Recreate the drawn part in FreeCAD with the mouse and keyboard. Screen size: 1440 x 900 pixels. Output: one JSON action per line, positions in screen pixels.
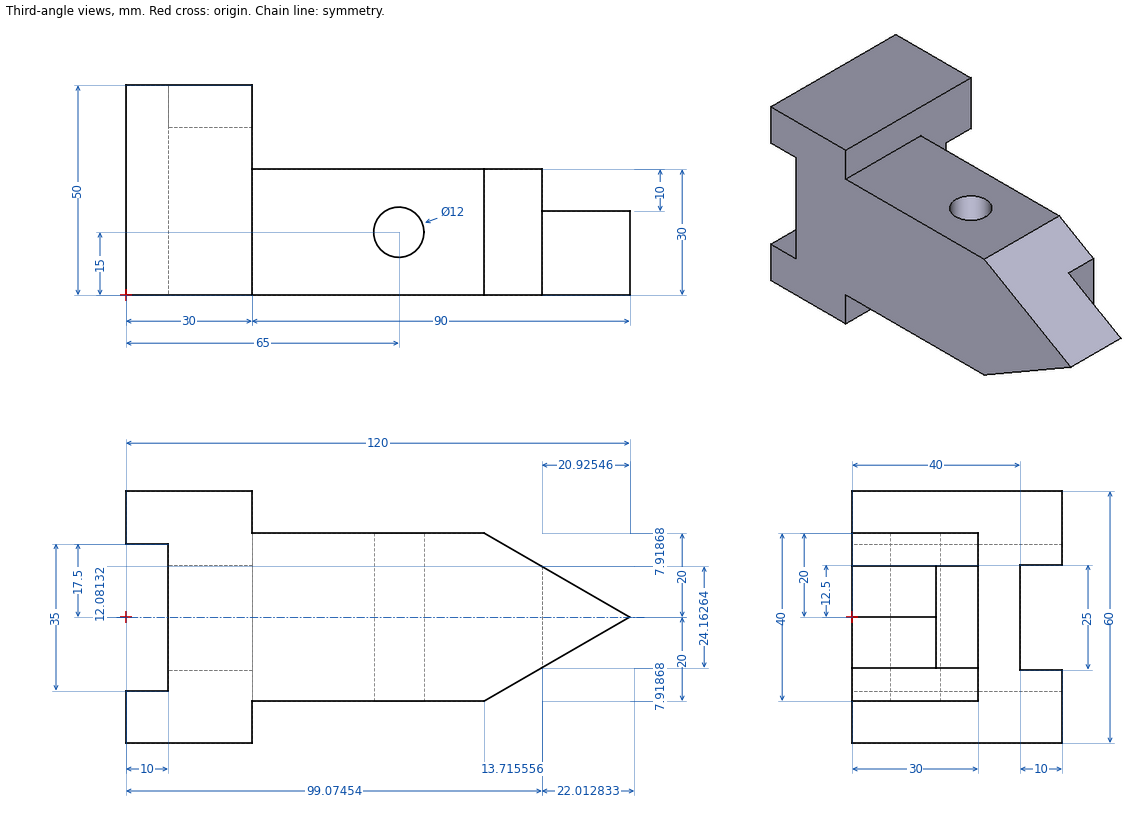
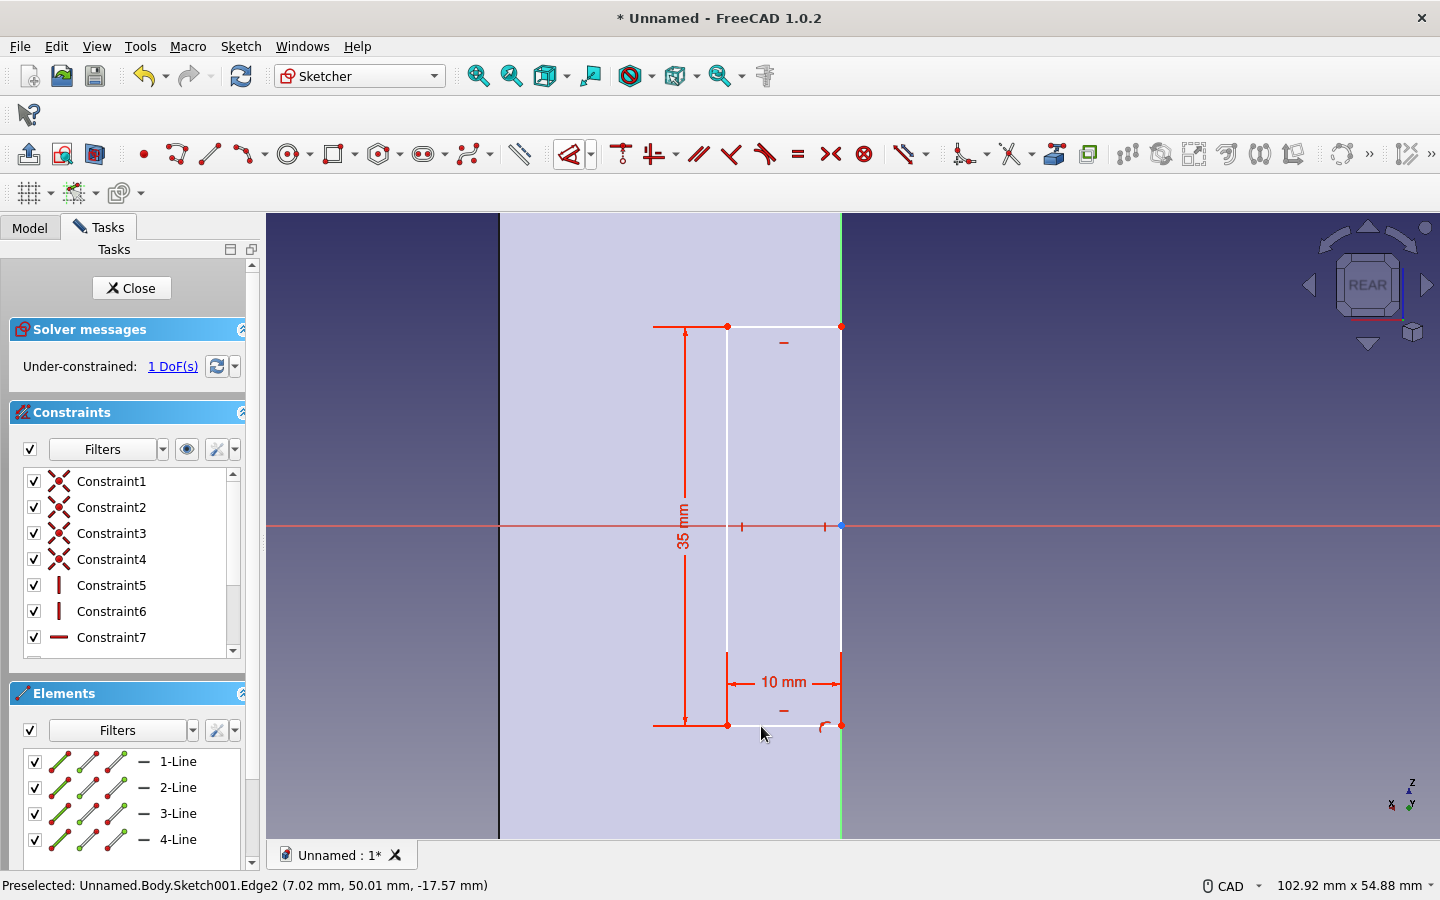
{"action": "left_click", "coordinate": [727, 327]}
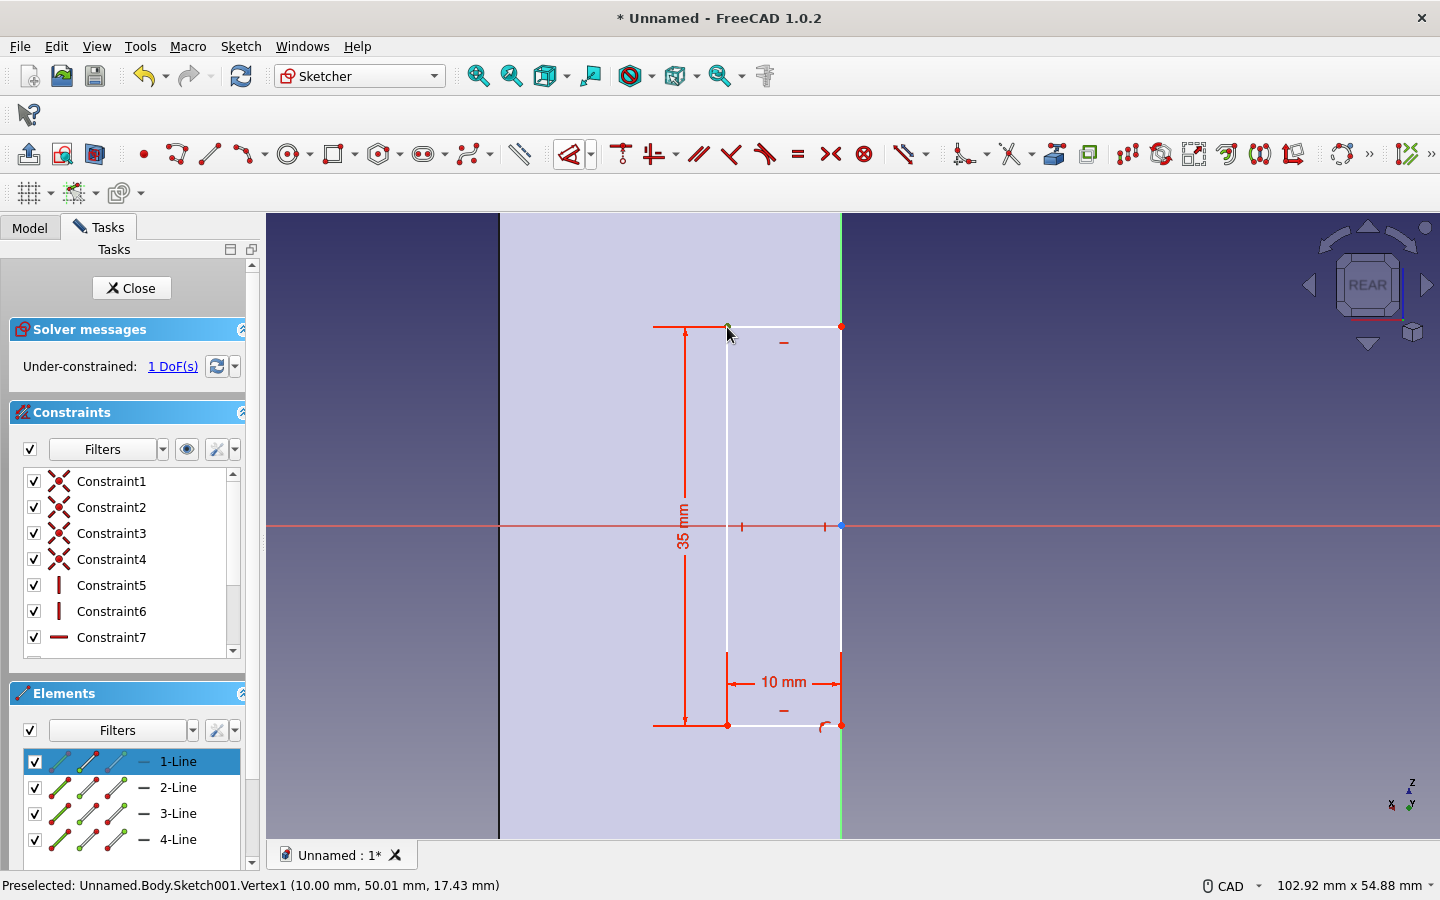
{"action": "left_click", "coordinate": [590, 154]}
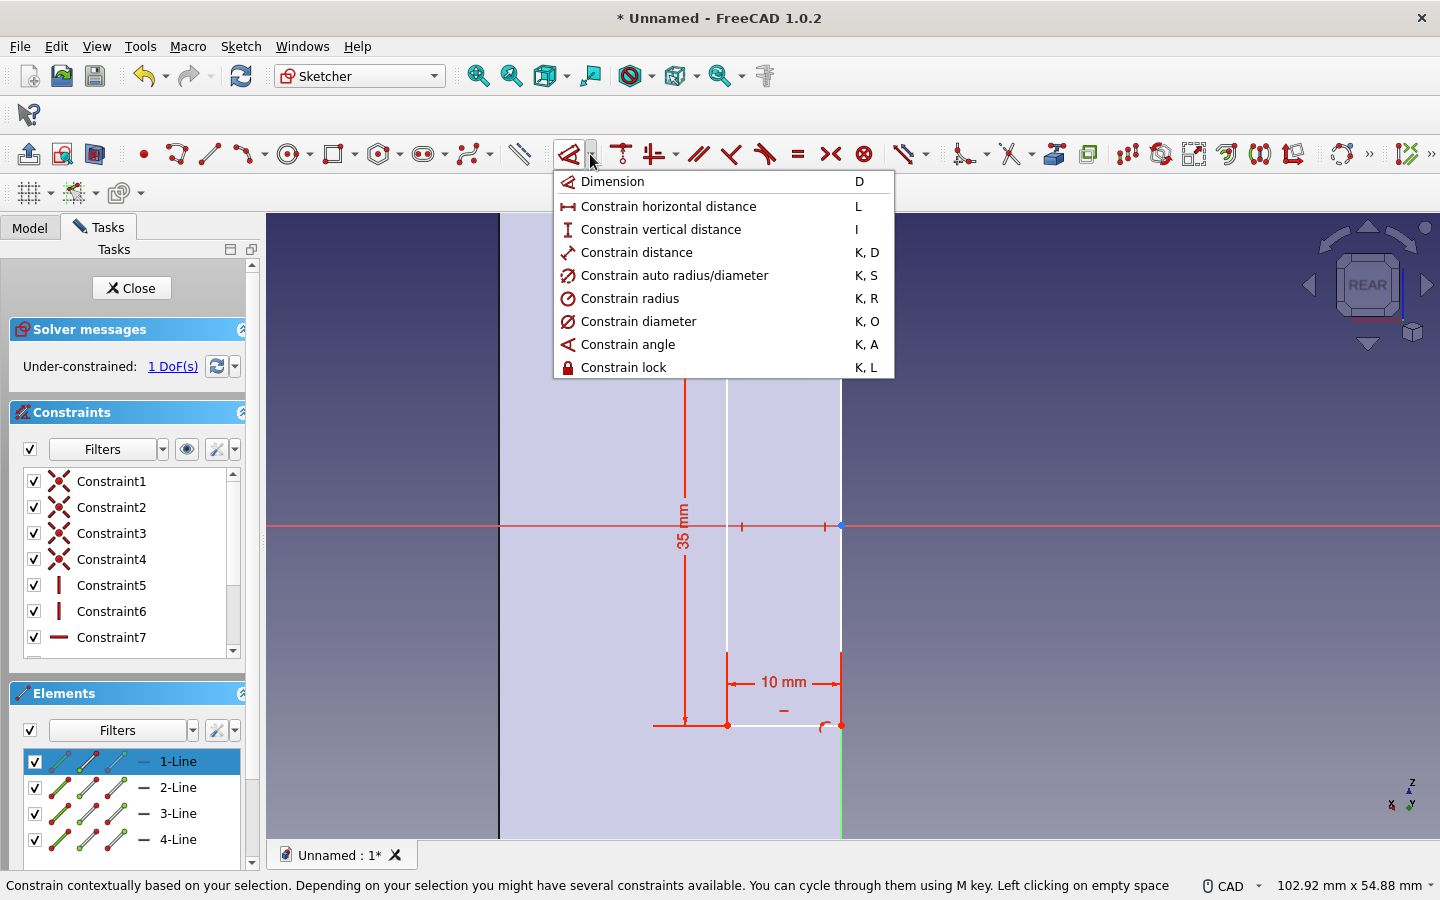
{"action": "left_click", "coordinate": [724, 230]}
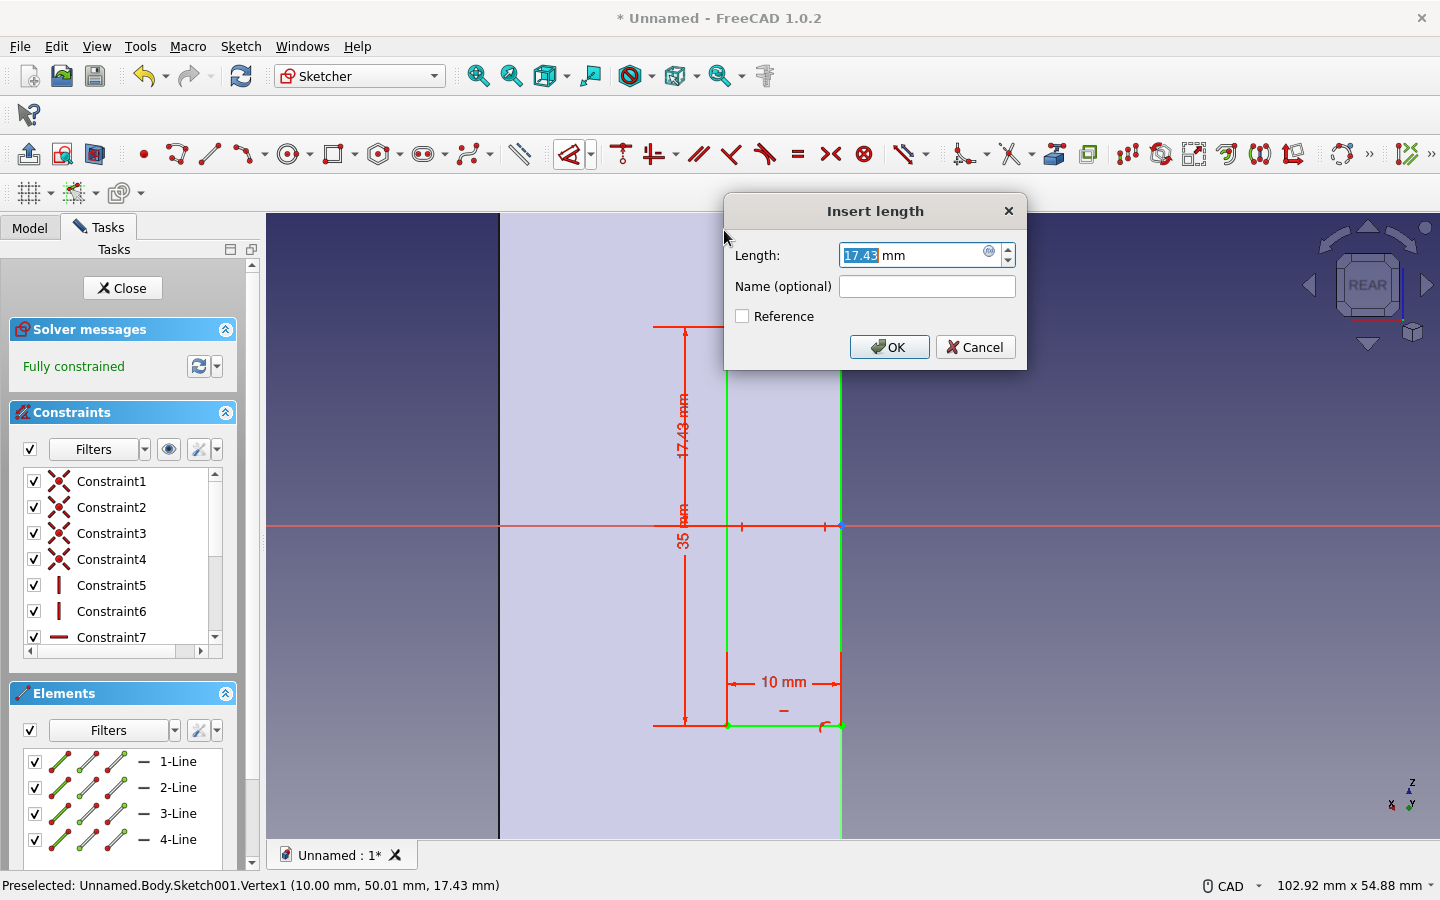
{"action": "type", "text": "17.5"}
{"action": "key", "text": "Return"}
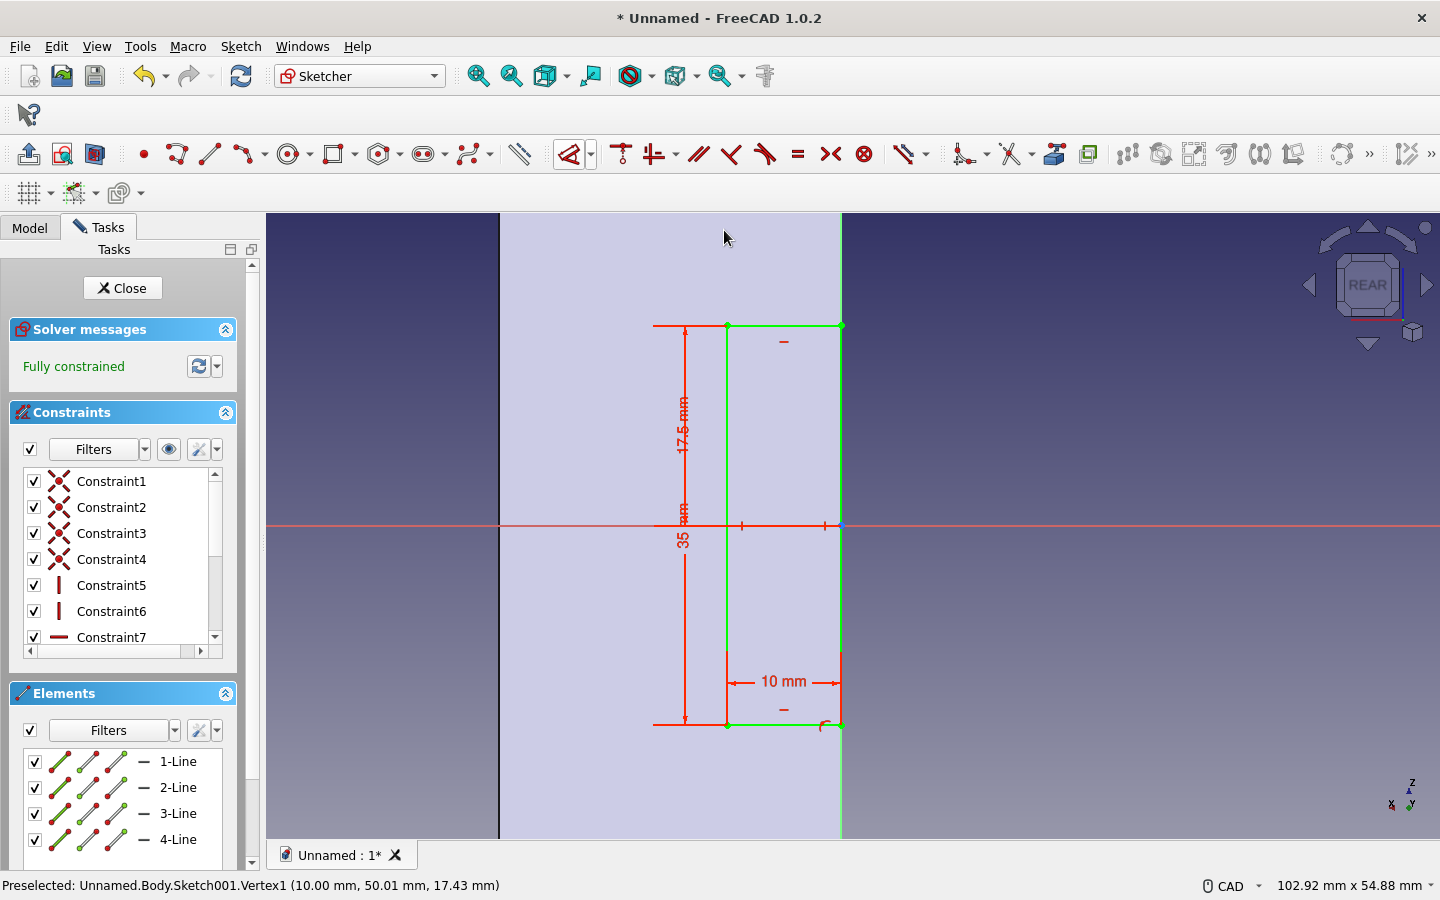
{"action": "left_click", "coordinate": [123, 288]}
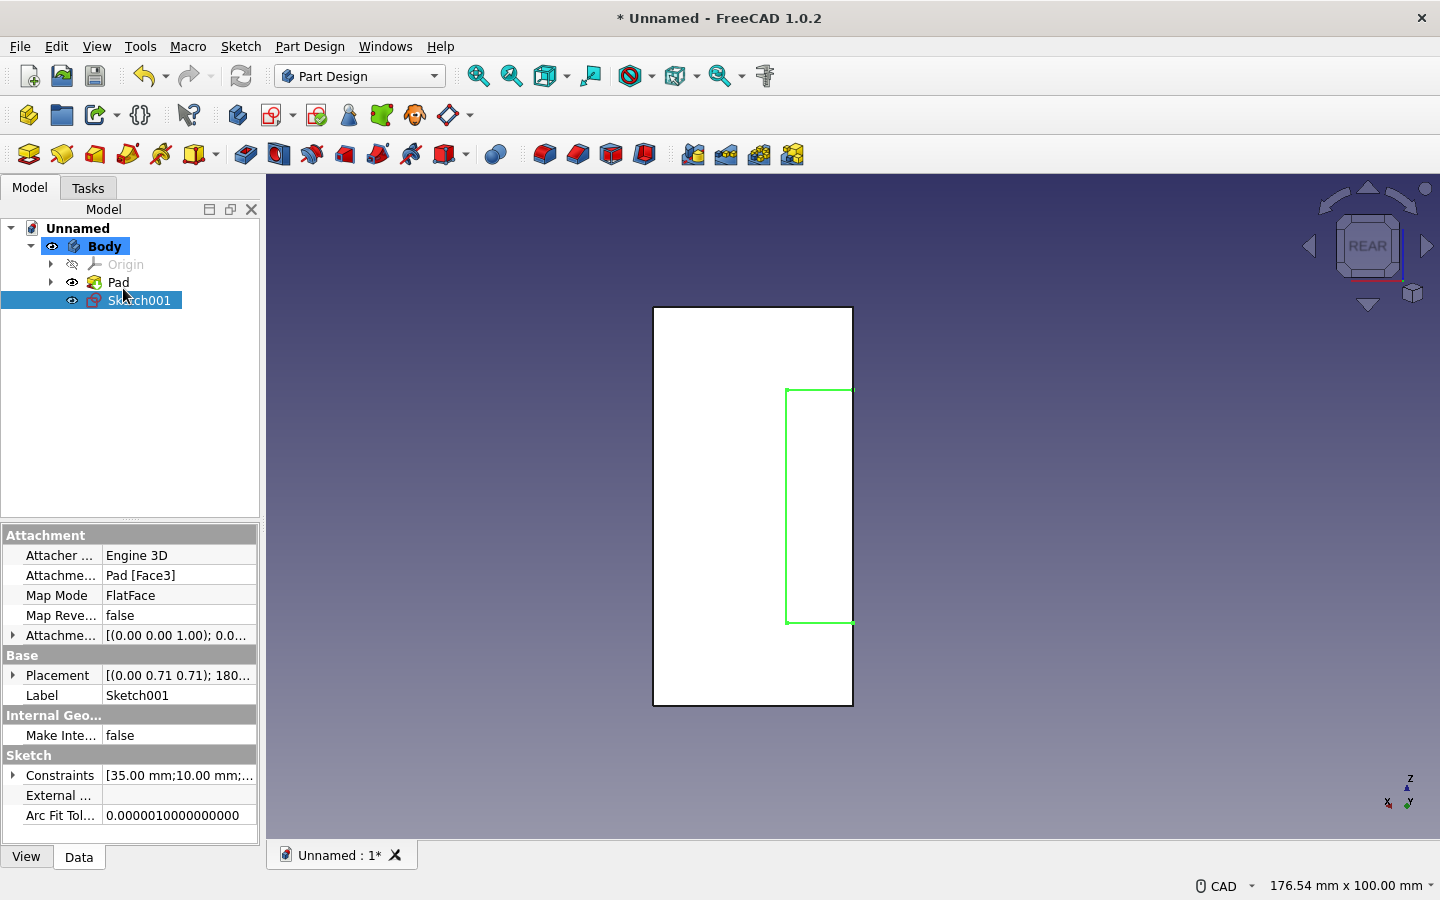
{"action": "left_click", "coordinate": [246, 154]}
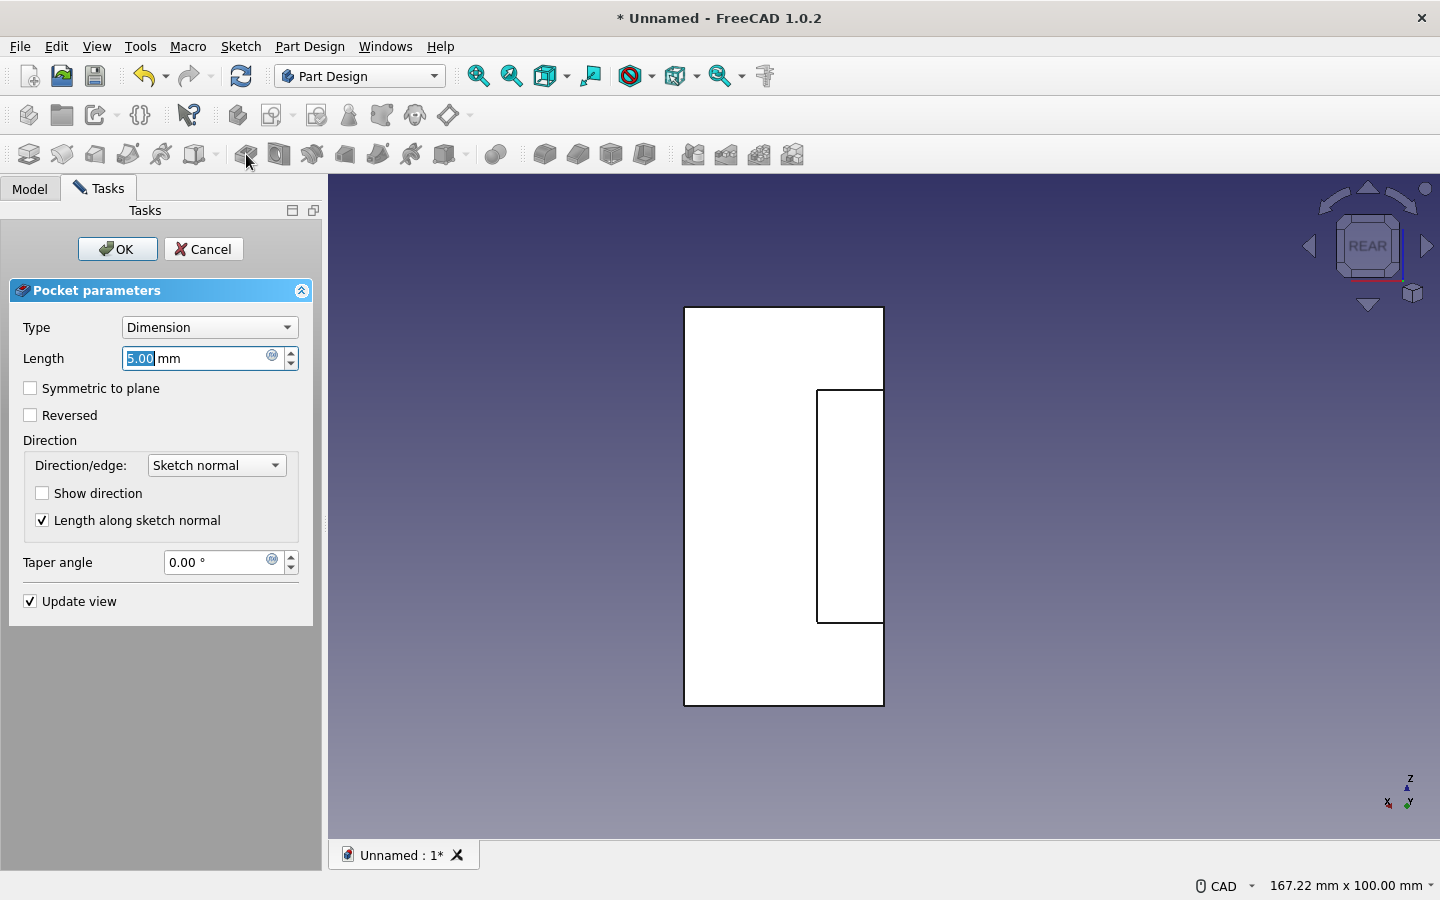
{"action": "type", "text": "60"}
{"action": "key", "text": "Tab"}